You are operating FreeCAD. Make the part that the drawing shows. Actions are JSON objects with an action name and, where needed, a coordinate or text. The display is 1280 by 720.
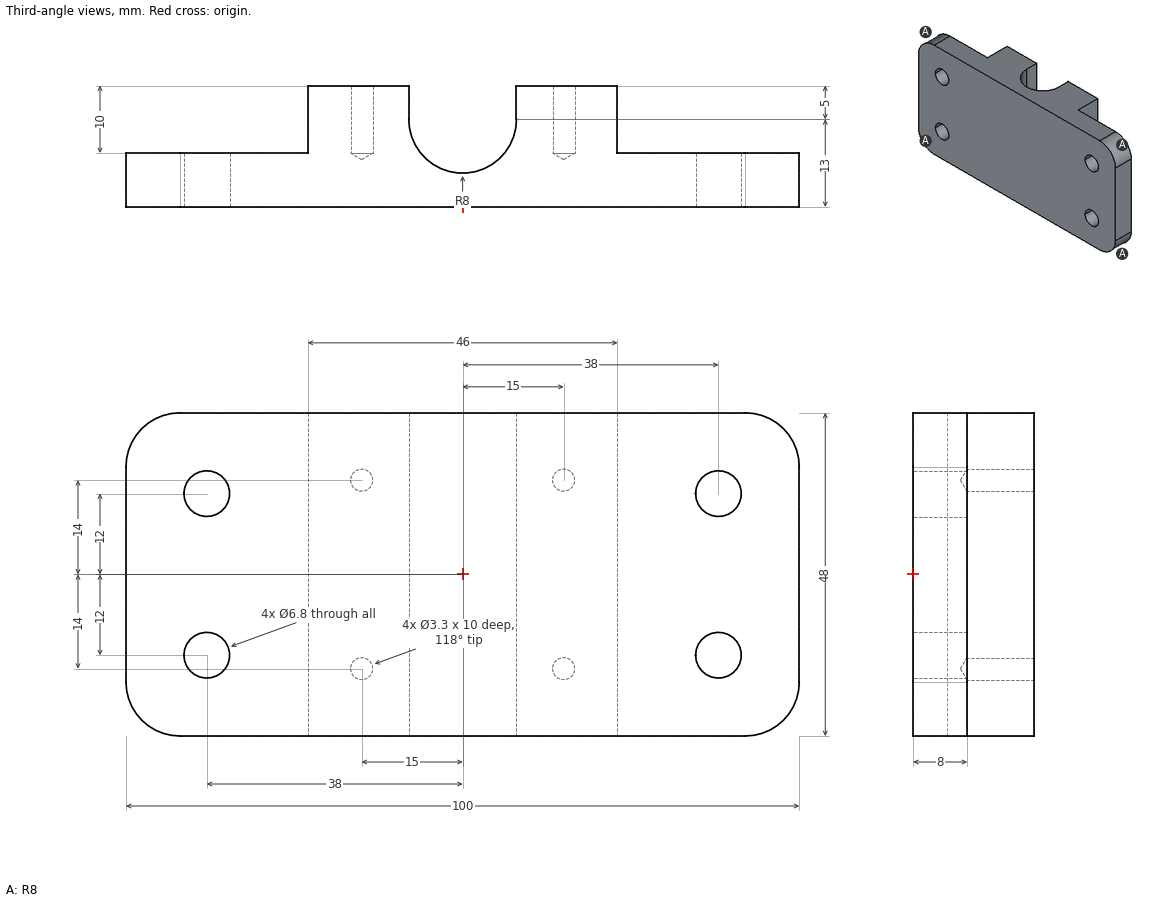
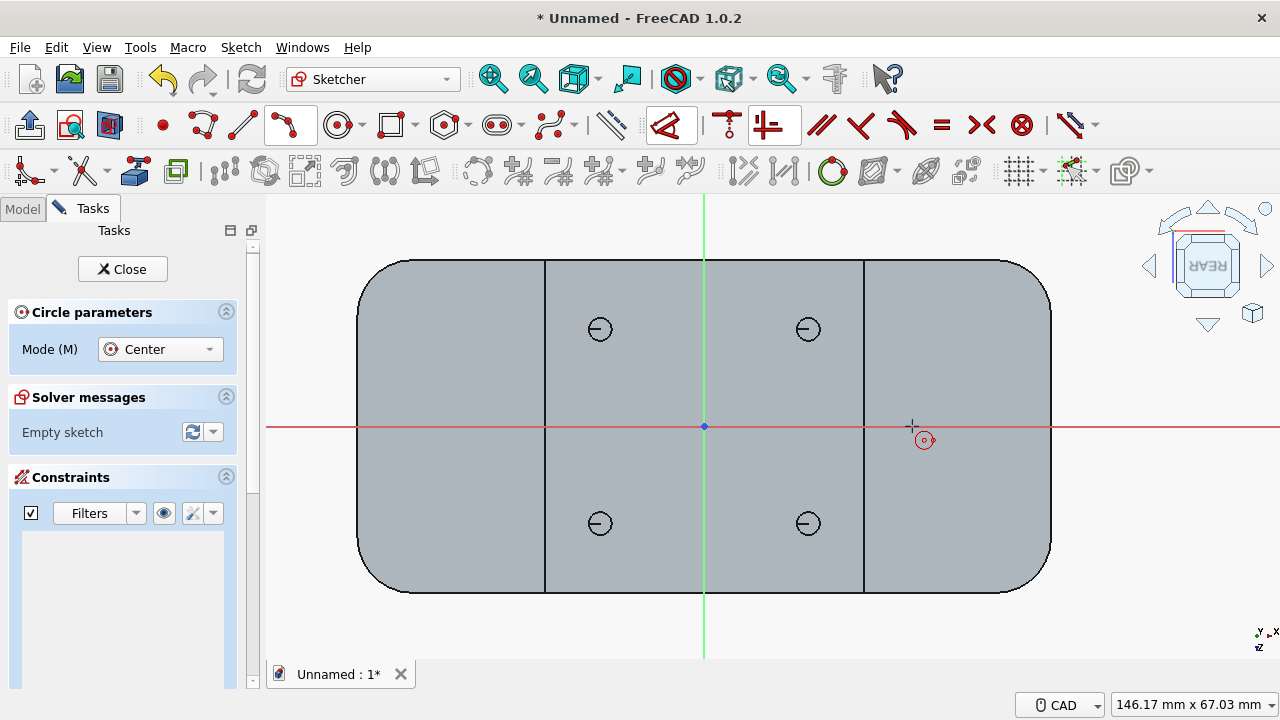
{"action": "left_click", "coordinate": [441, 343]}
{"action": "left_click", "coordinate": [457, 327]}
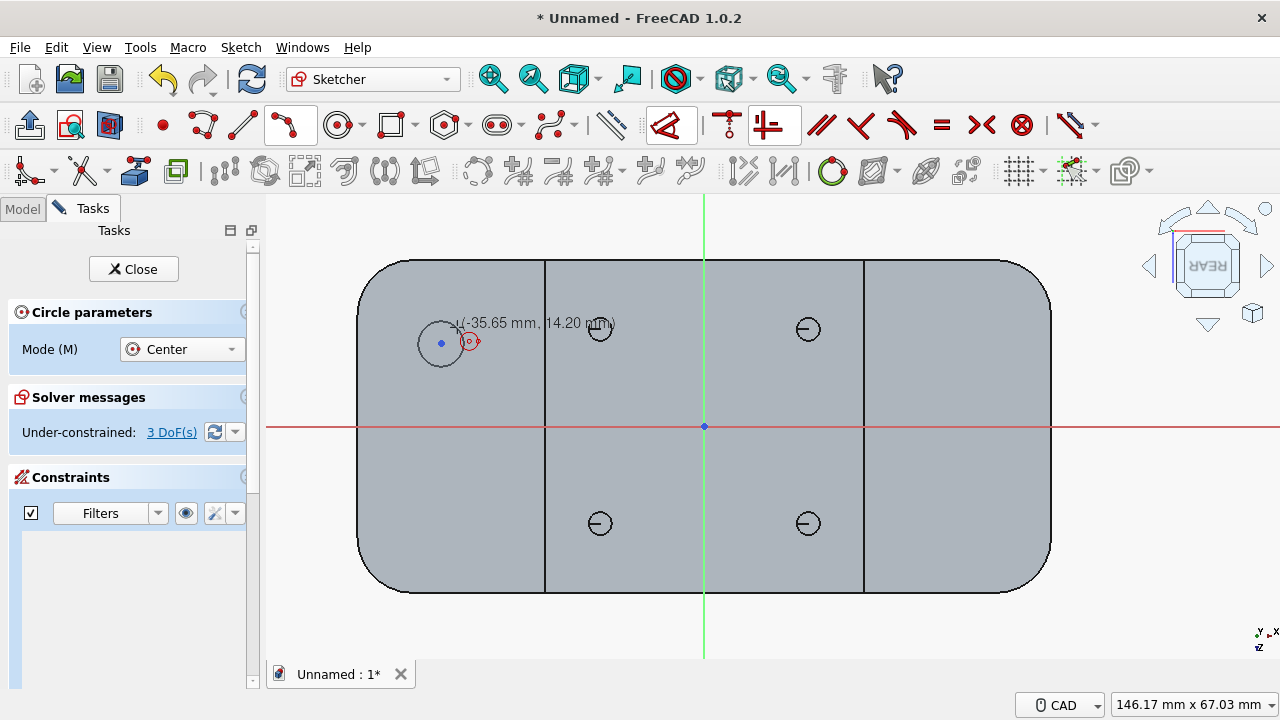
{"action": "left_click", "coordinate": [441, 510]}
{"action": "left_click", "coordinate": [457, 493]}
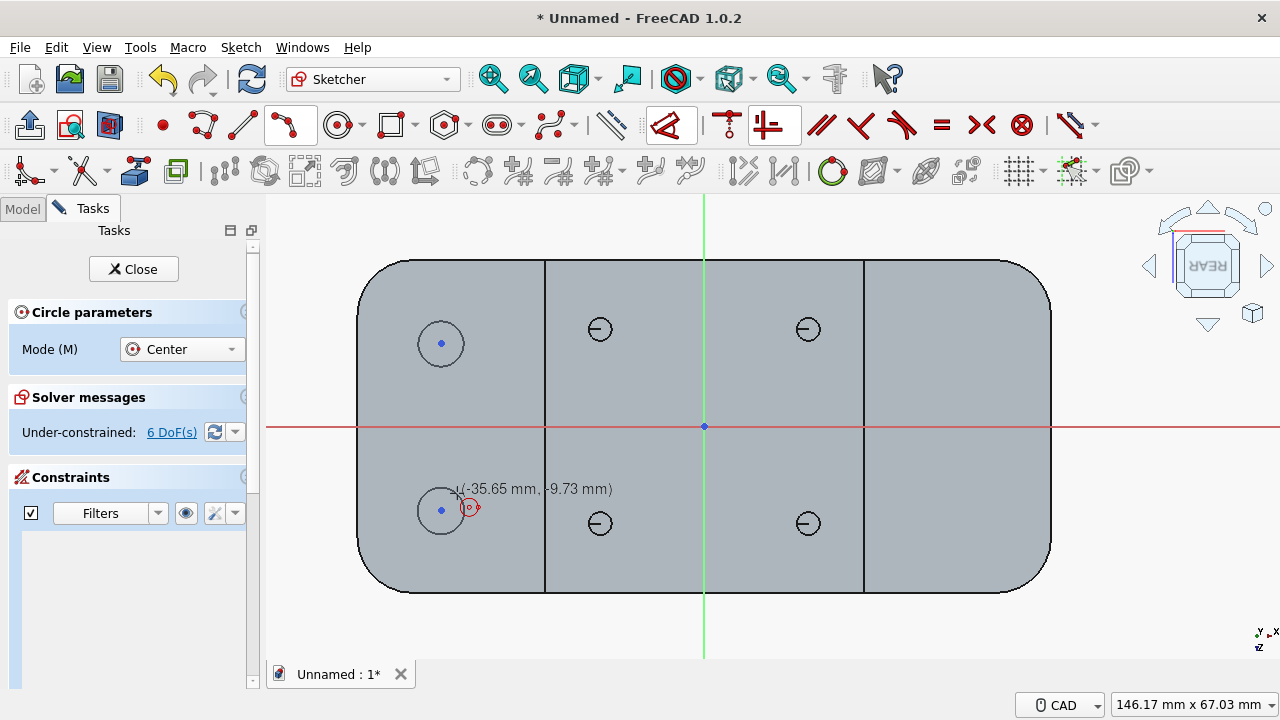
{"action": "left_click", "coordinate": [968, 510]}
{"action": "left_click", "coordinate": [985, 493]}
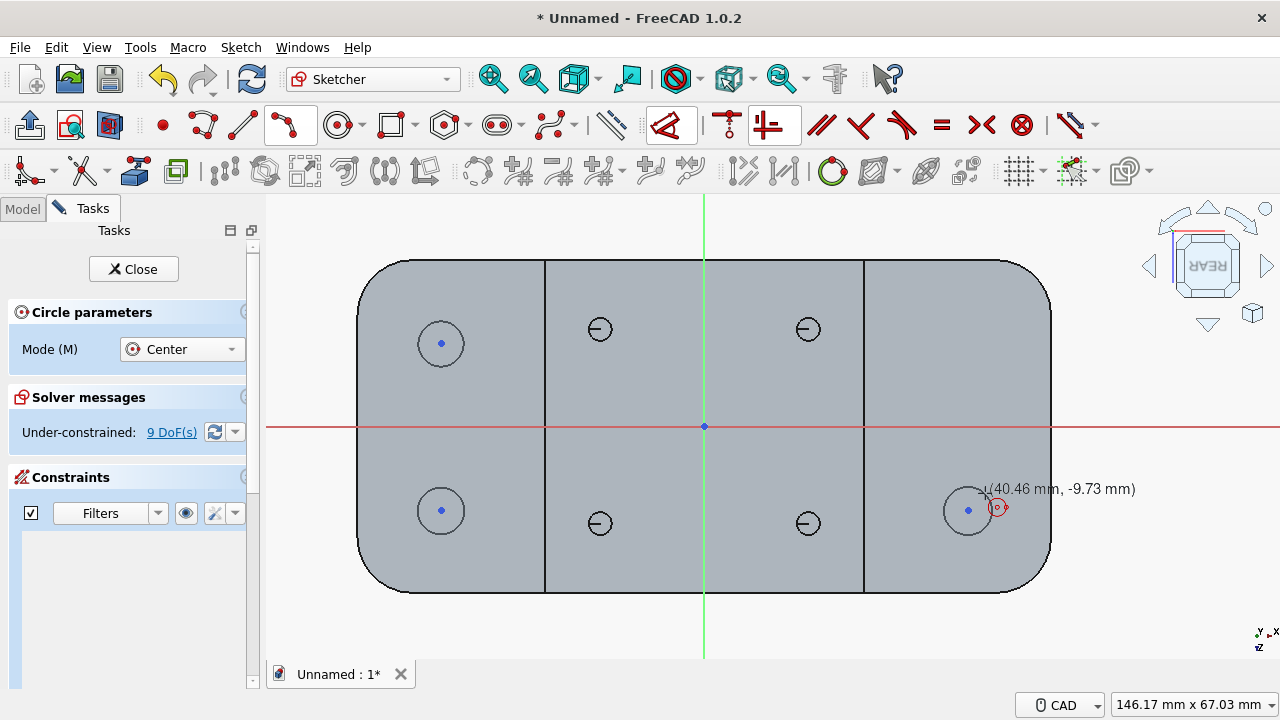
{"action": "left_click", "coordinate": [968, 343]}
{"action": "left_click", "coordinate": [985, 327]}
{"action": "key", "text": "Escape"}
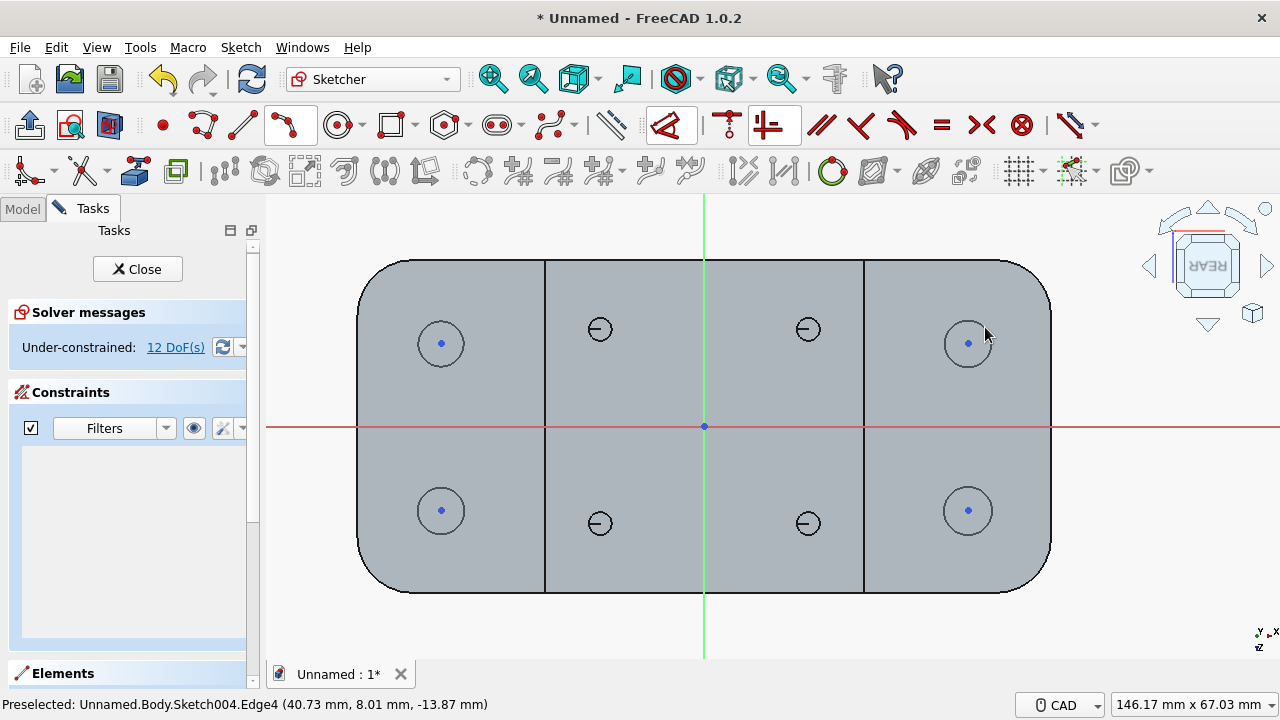
{"action": "left_click", "coordinate": [457, 328]}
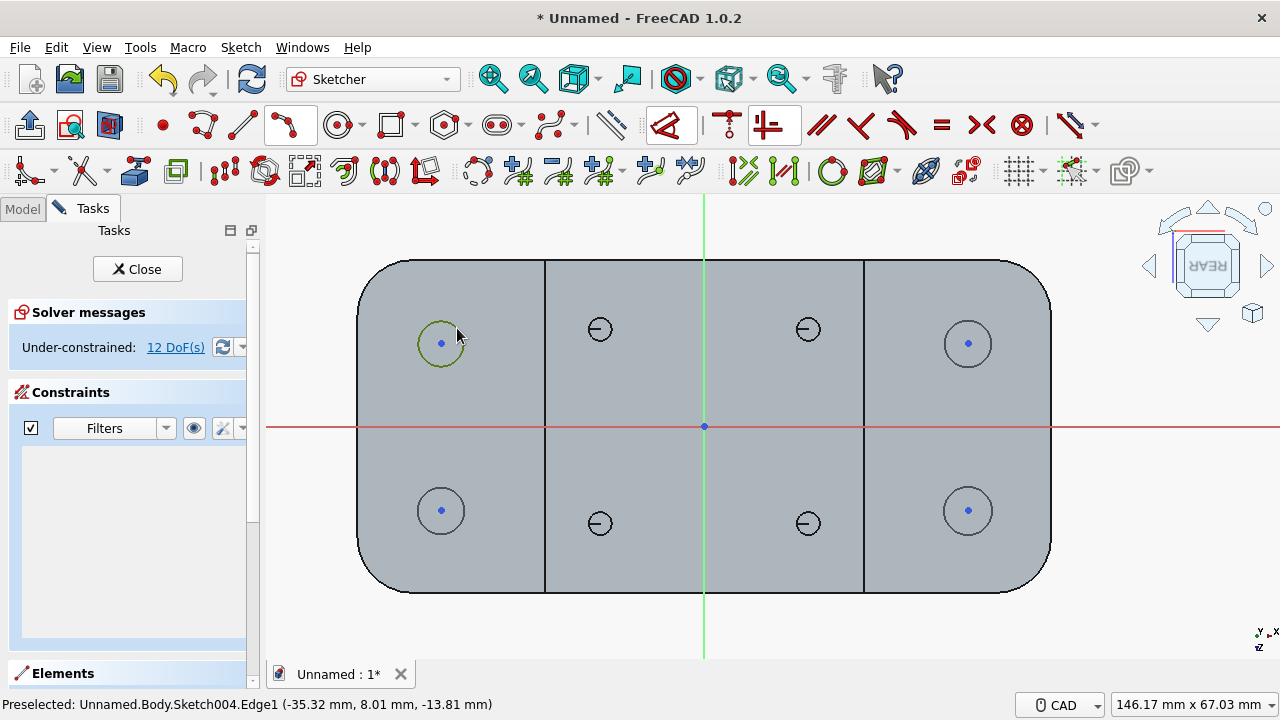
{"action": "left_click", "coordinate": [457, 494]}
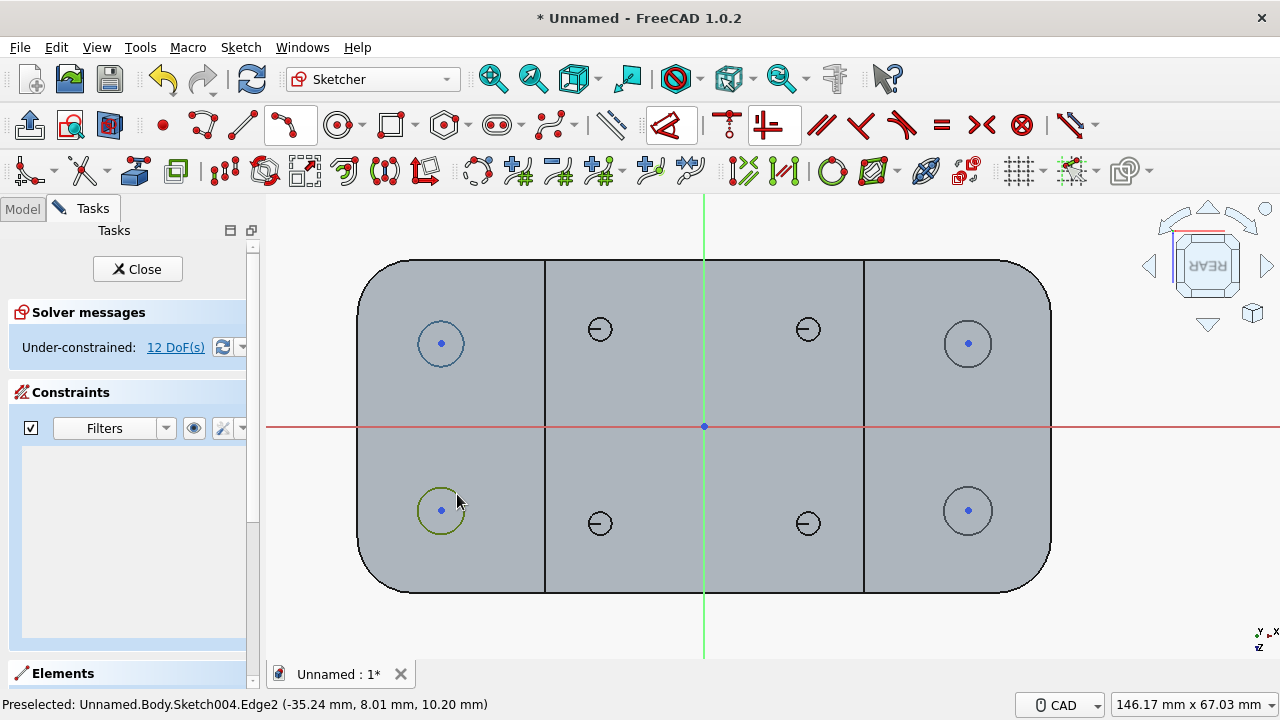
{"action": "left_click", "coordinate": [985, 494]}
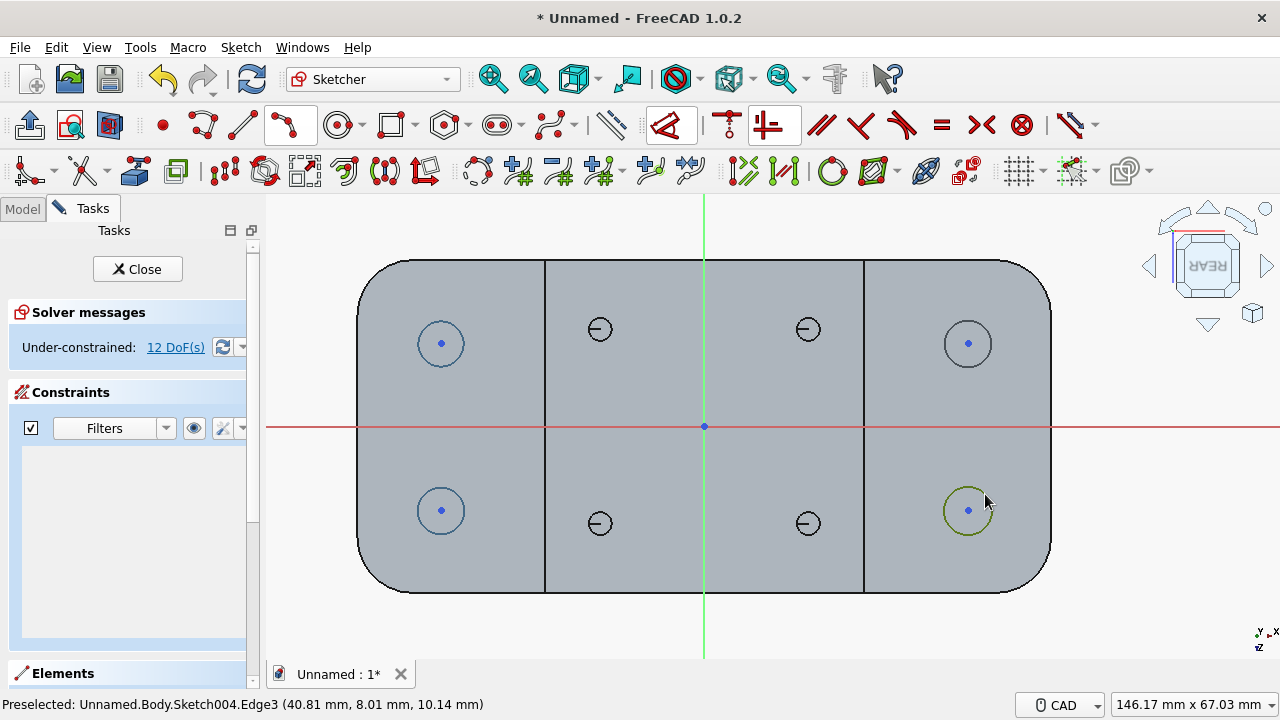
{"action": "left_click", "coordinate": [984, 327]}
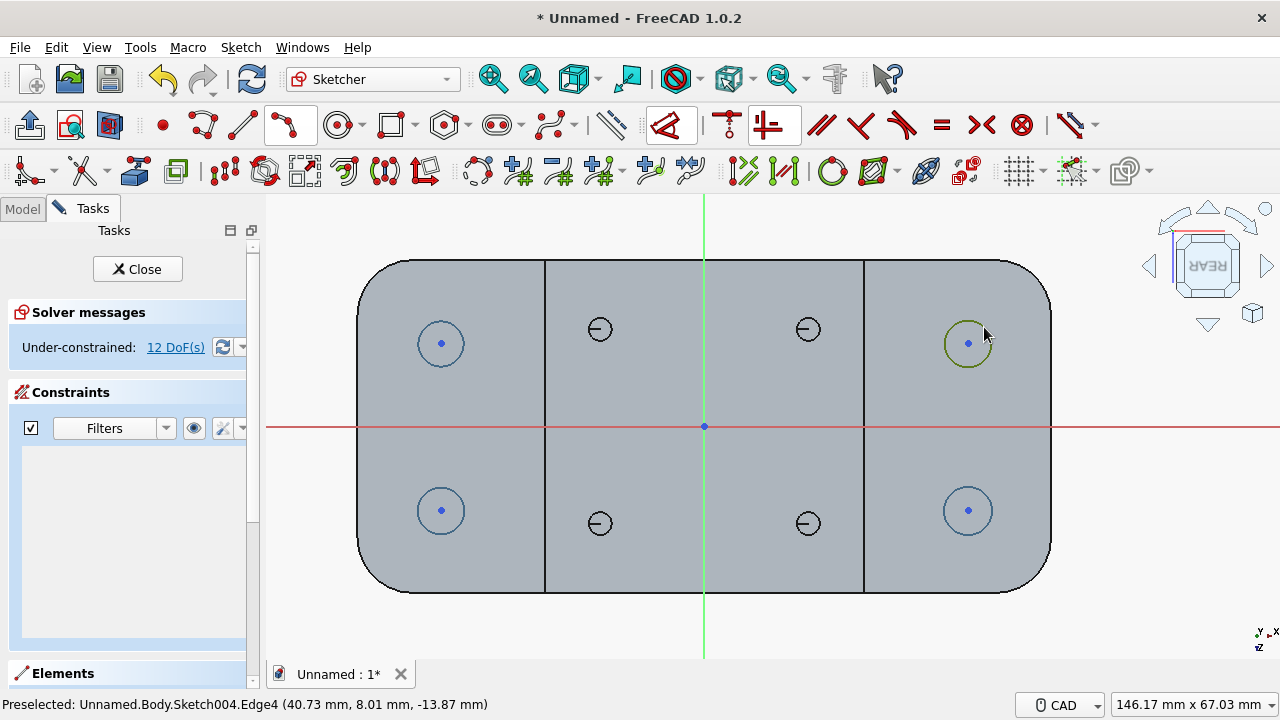
{"action": "left_click", "coordinate": [942, 126]}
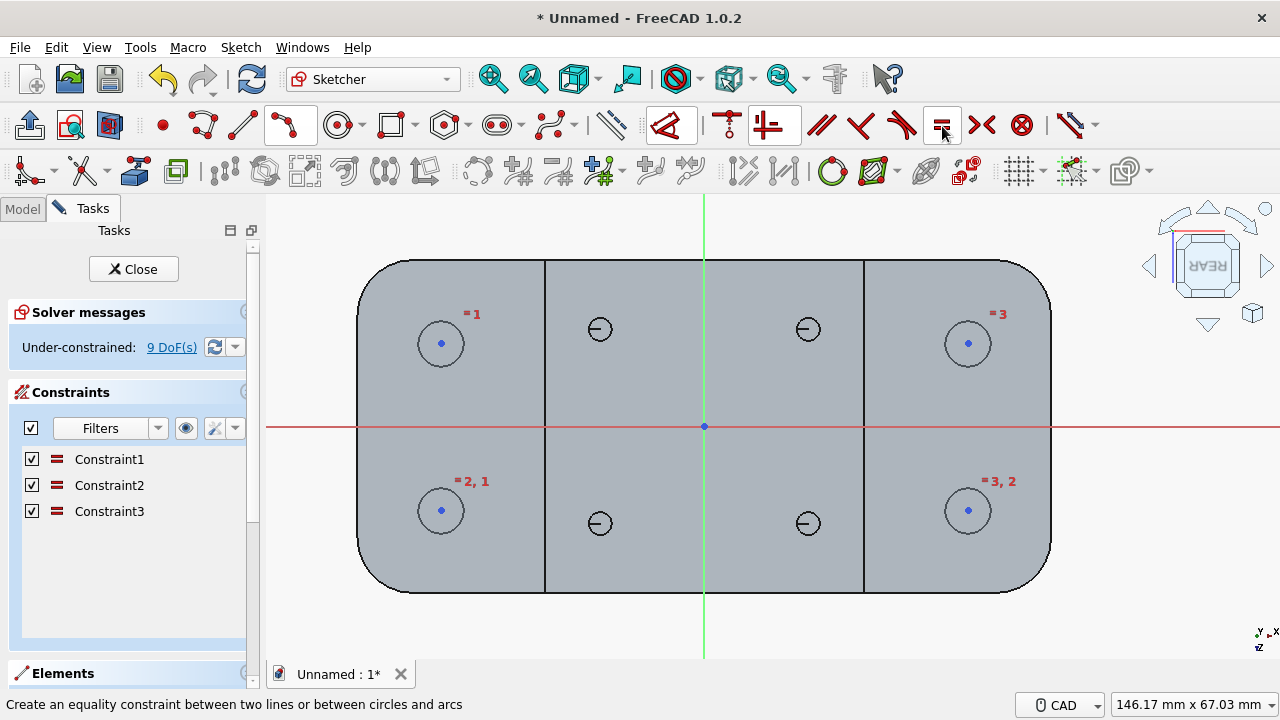
{"action": "left_click", "coordinate": [441, 344]}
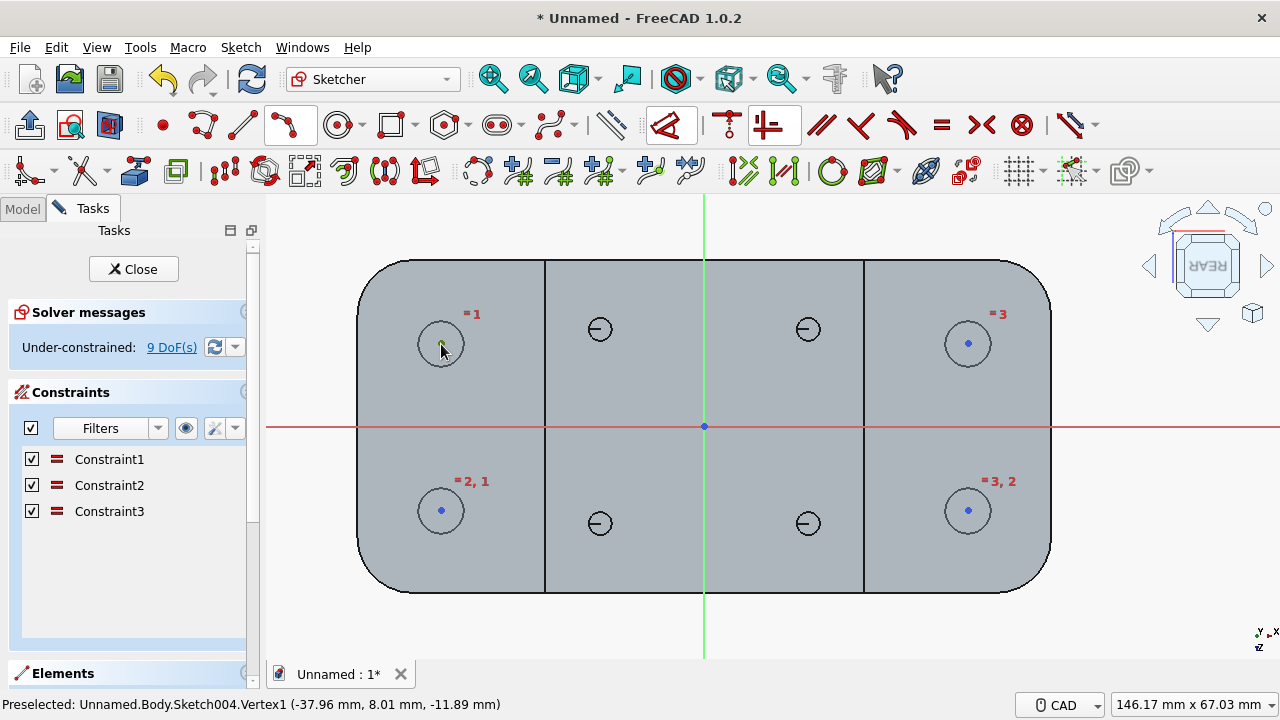
{"action": "left_click", "coordinate": [441, 511]}